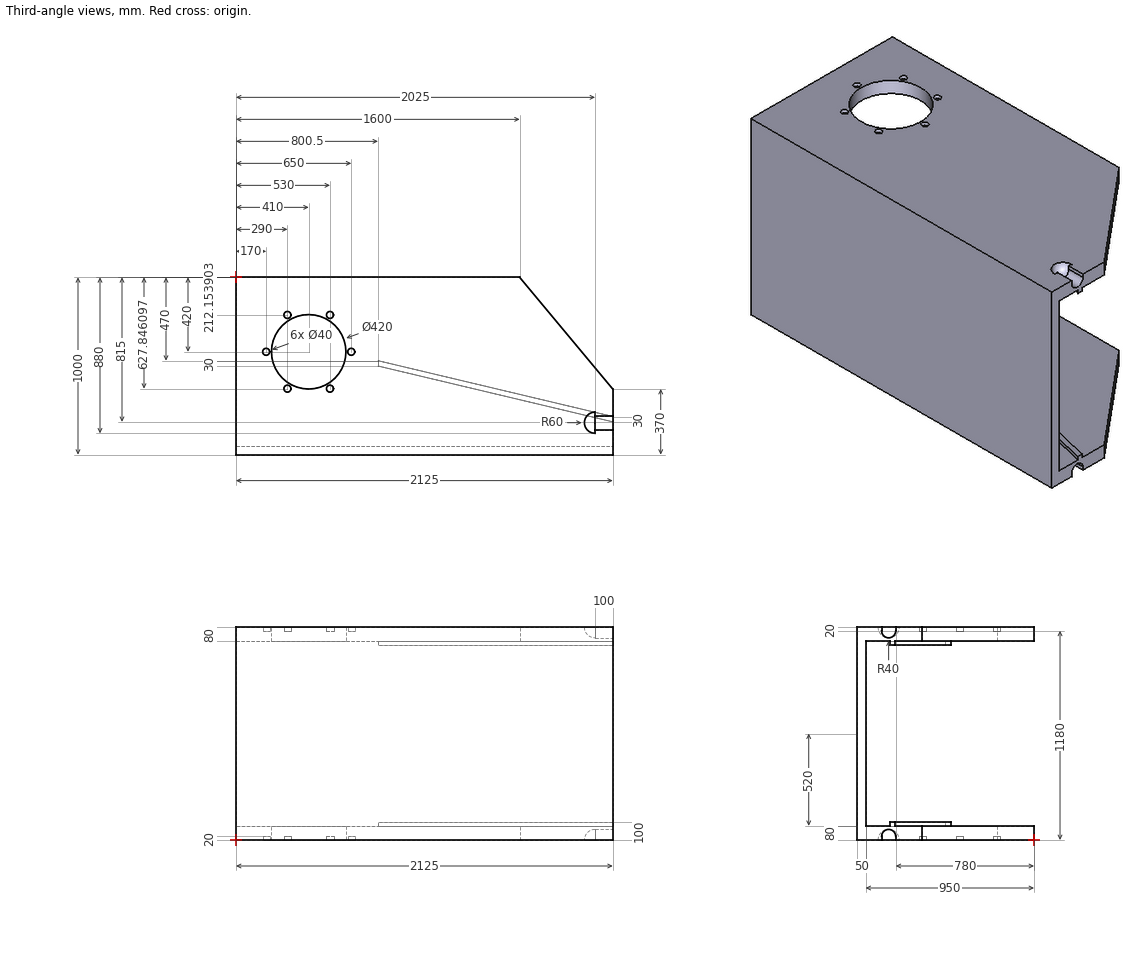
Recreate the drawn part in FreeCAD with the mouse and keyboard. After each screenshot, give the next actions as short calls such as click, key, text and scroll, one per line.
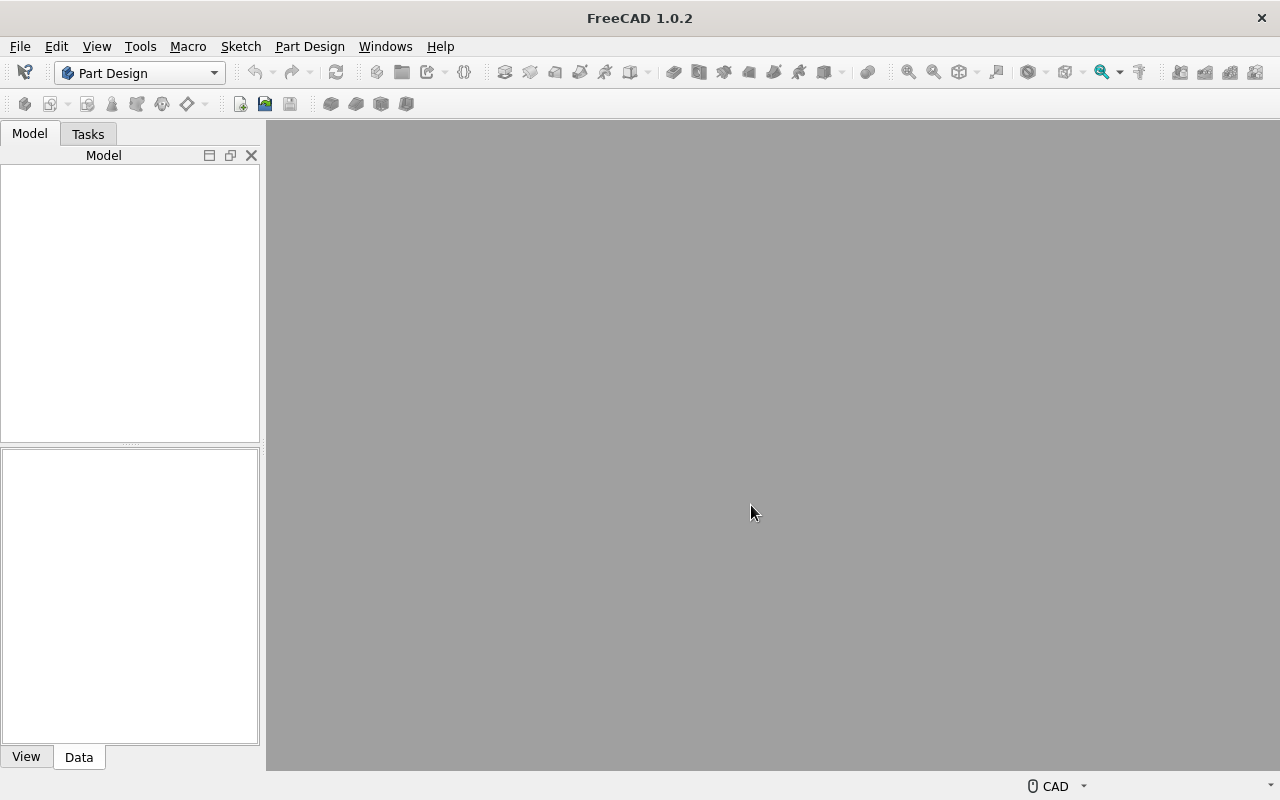
key(ctrl+n)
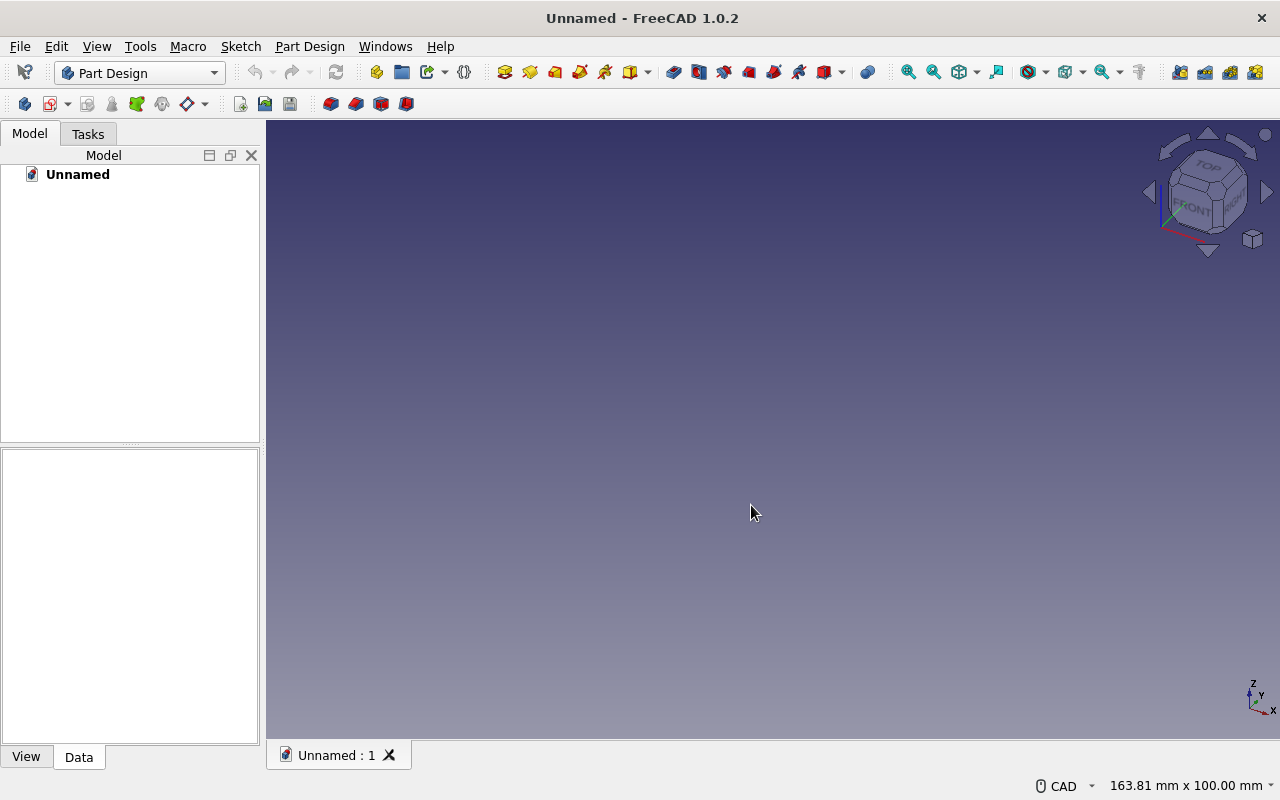
click(50, 104)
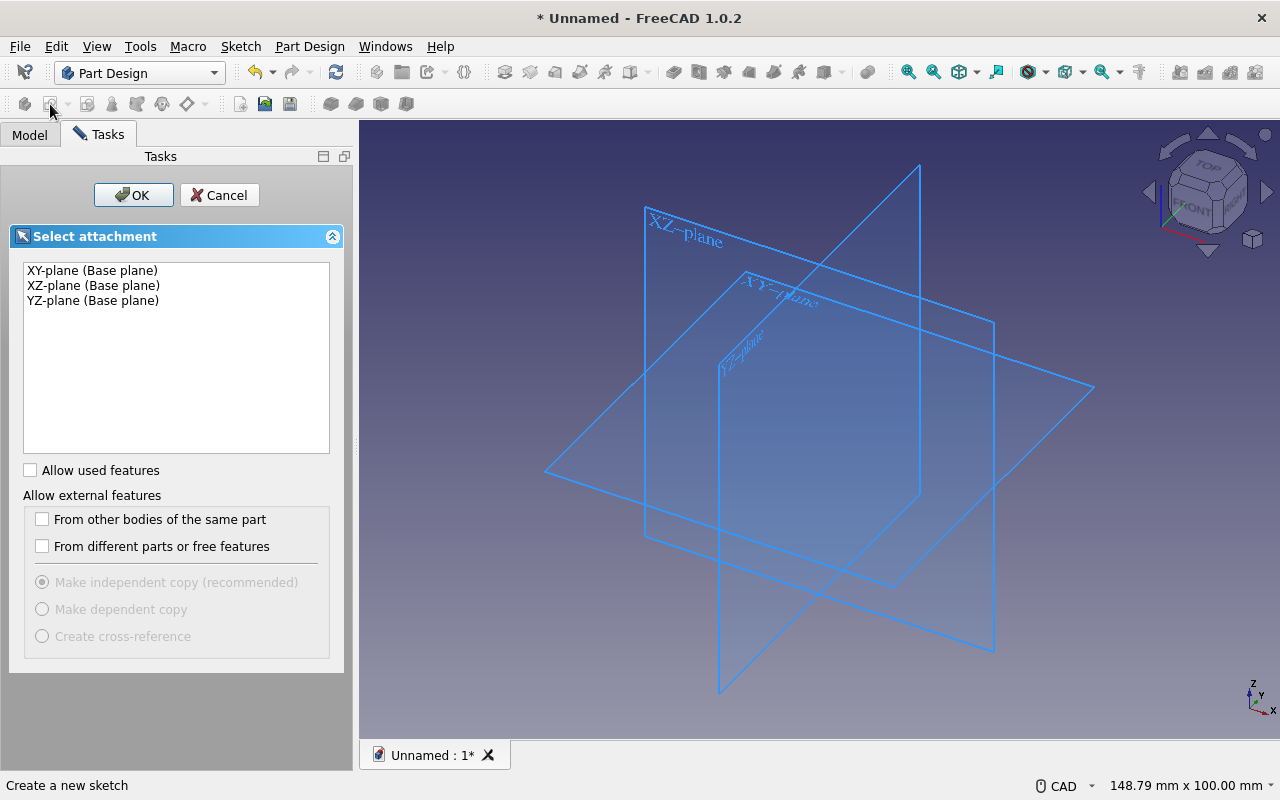
click(84, 270)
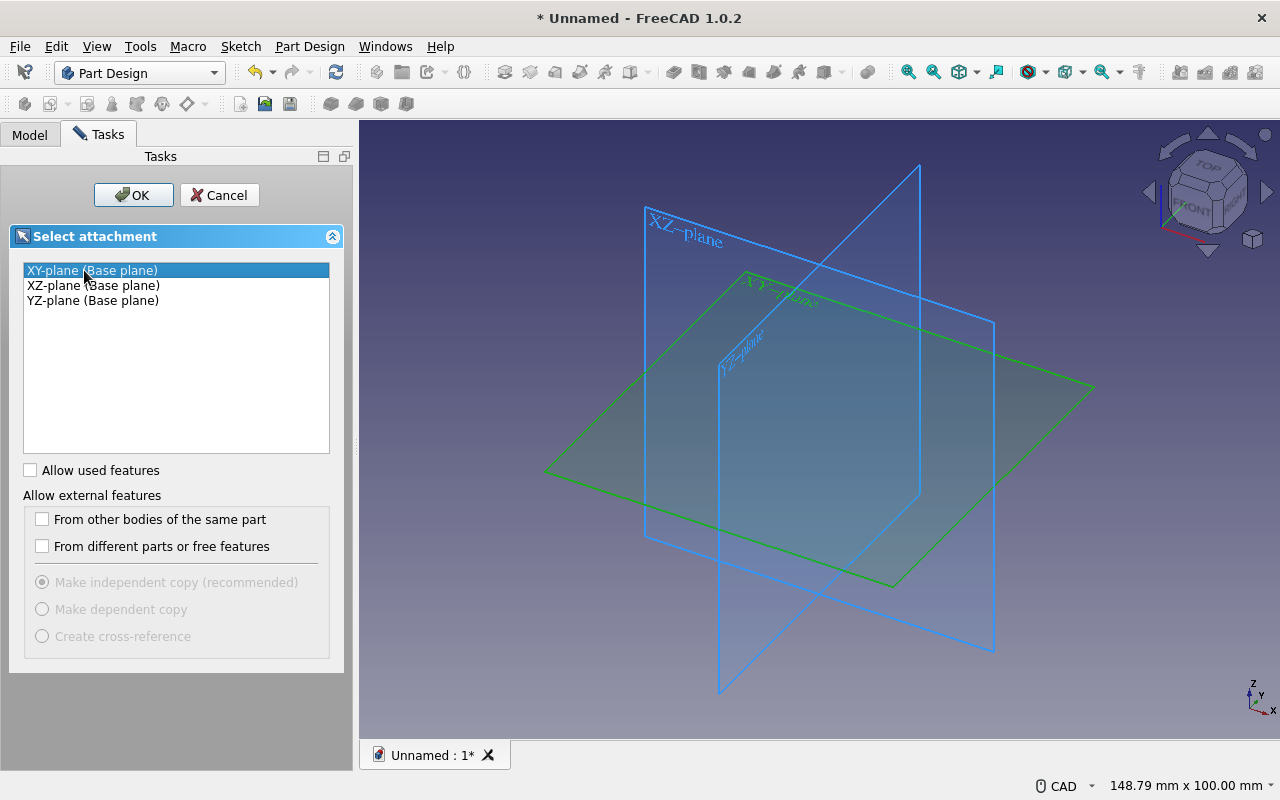
click(134, 195)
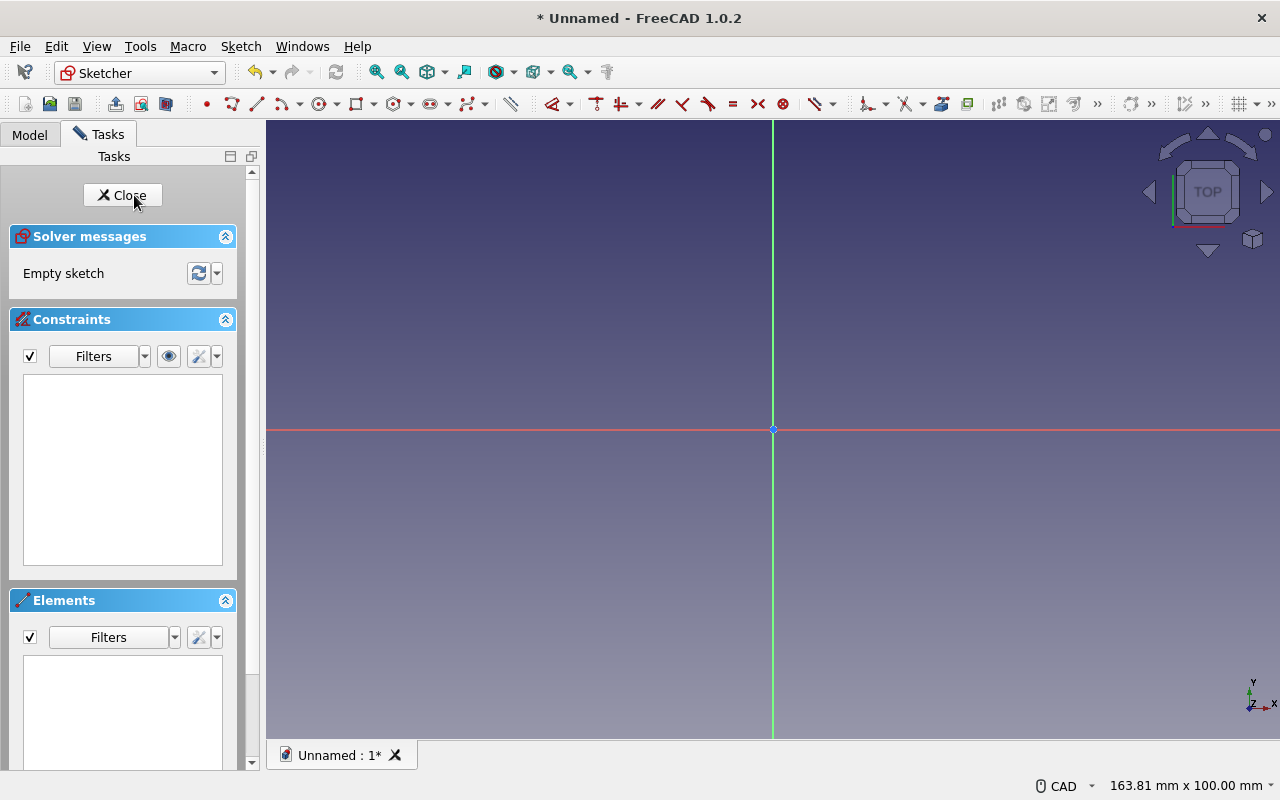
scroll(356, 267, down, 15)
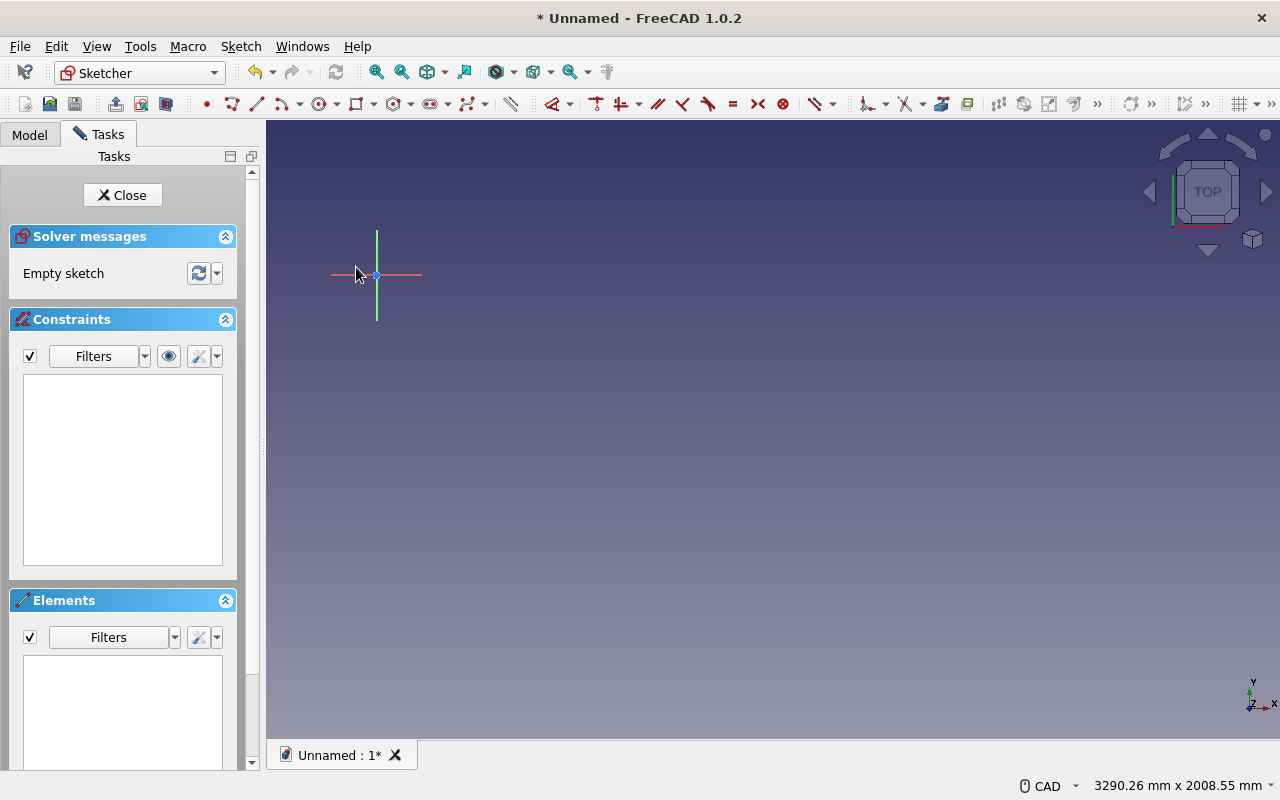
key(g)
key(m)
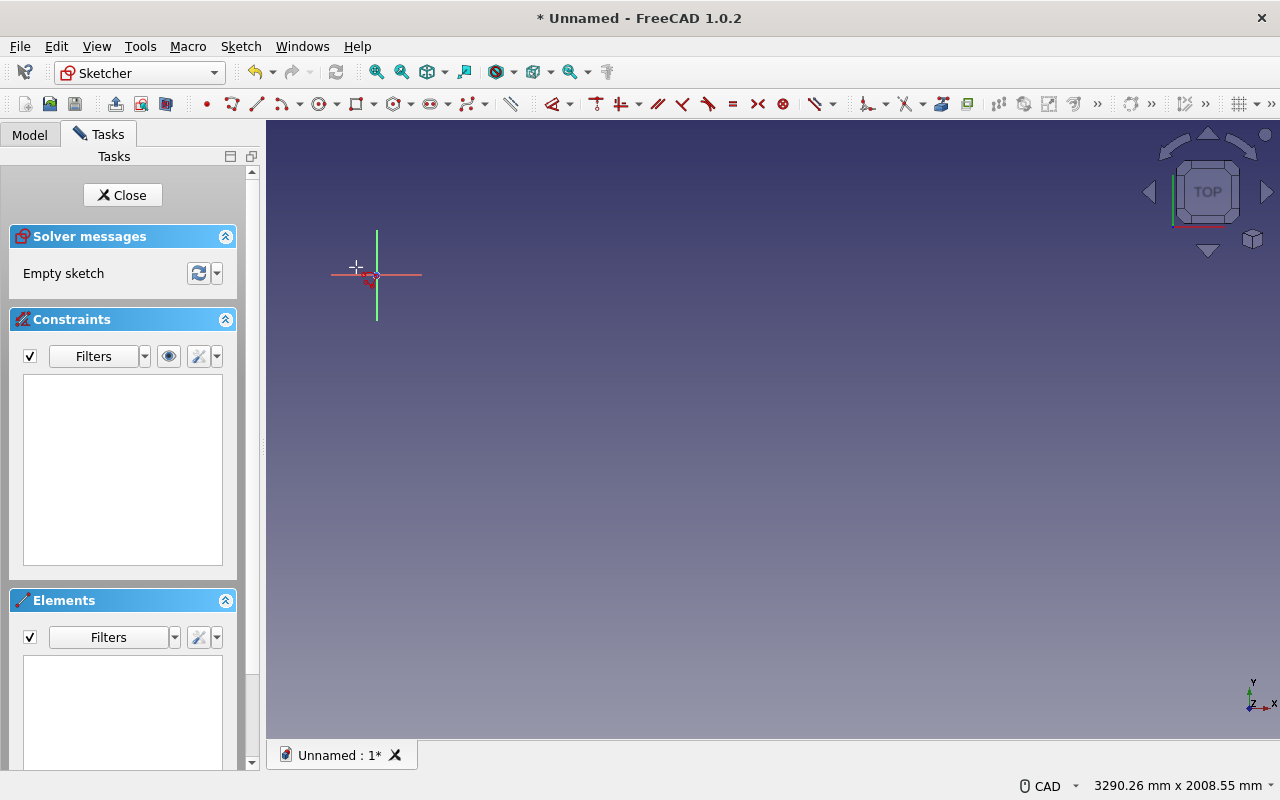
click(377, 275)
click(386, 583)
click(1032, 583)
click(1032, 469)
click(870, 284)
click(377, 275)
key(Escape)
key(Escape)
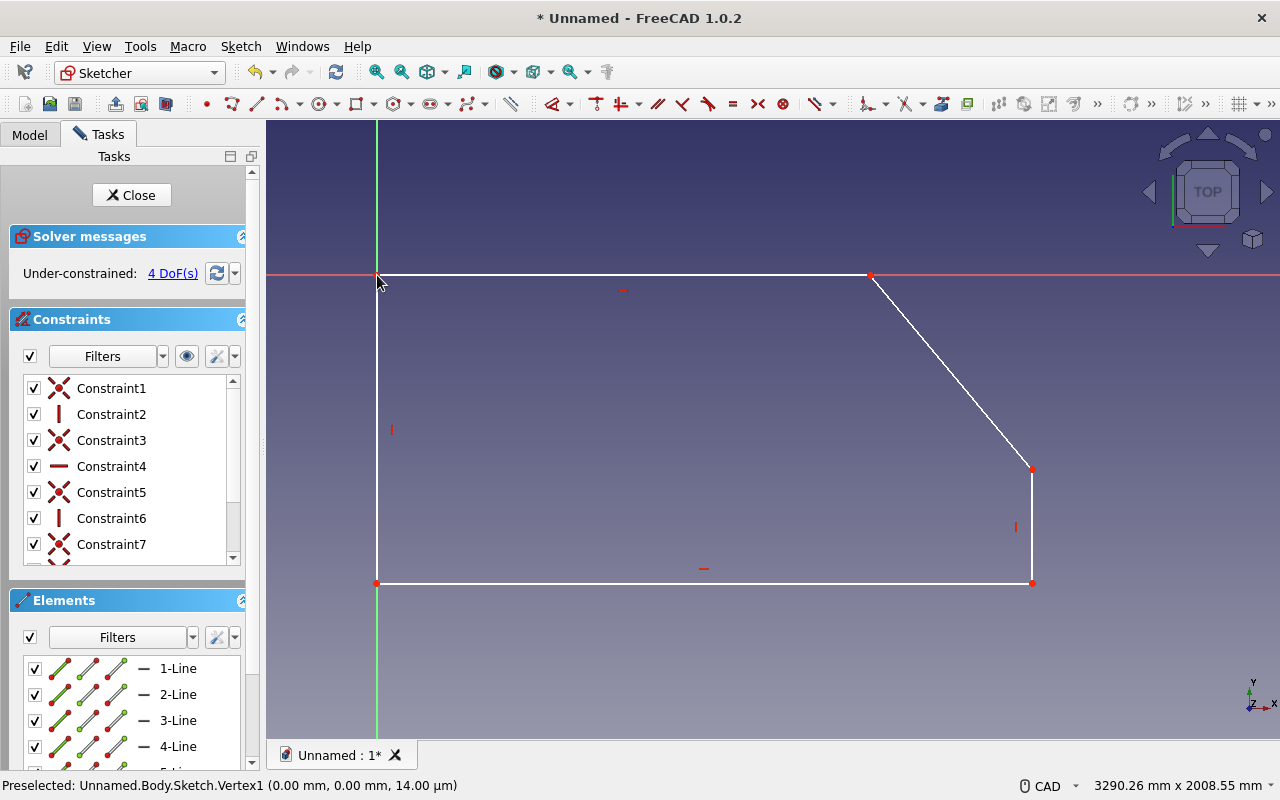
key(d)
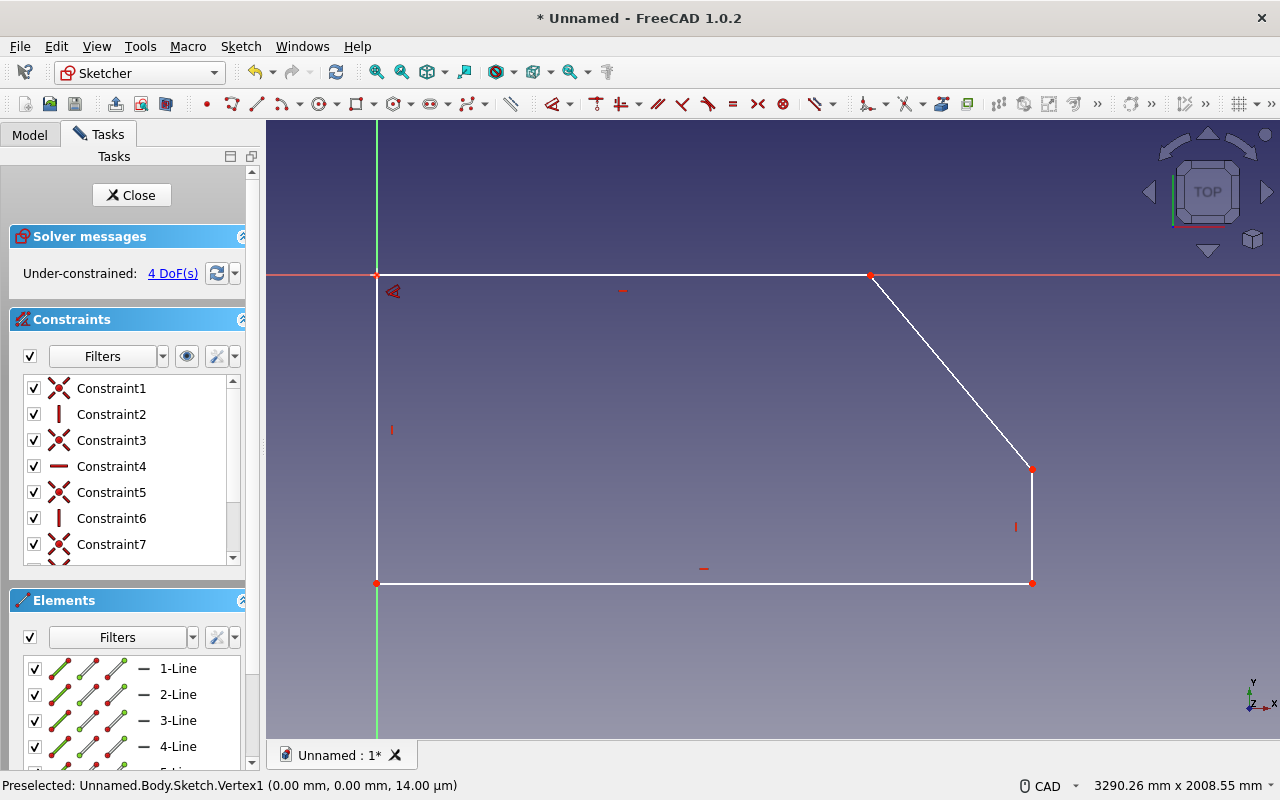
click(1032, 550)
click(1066, 527)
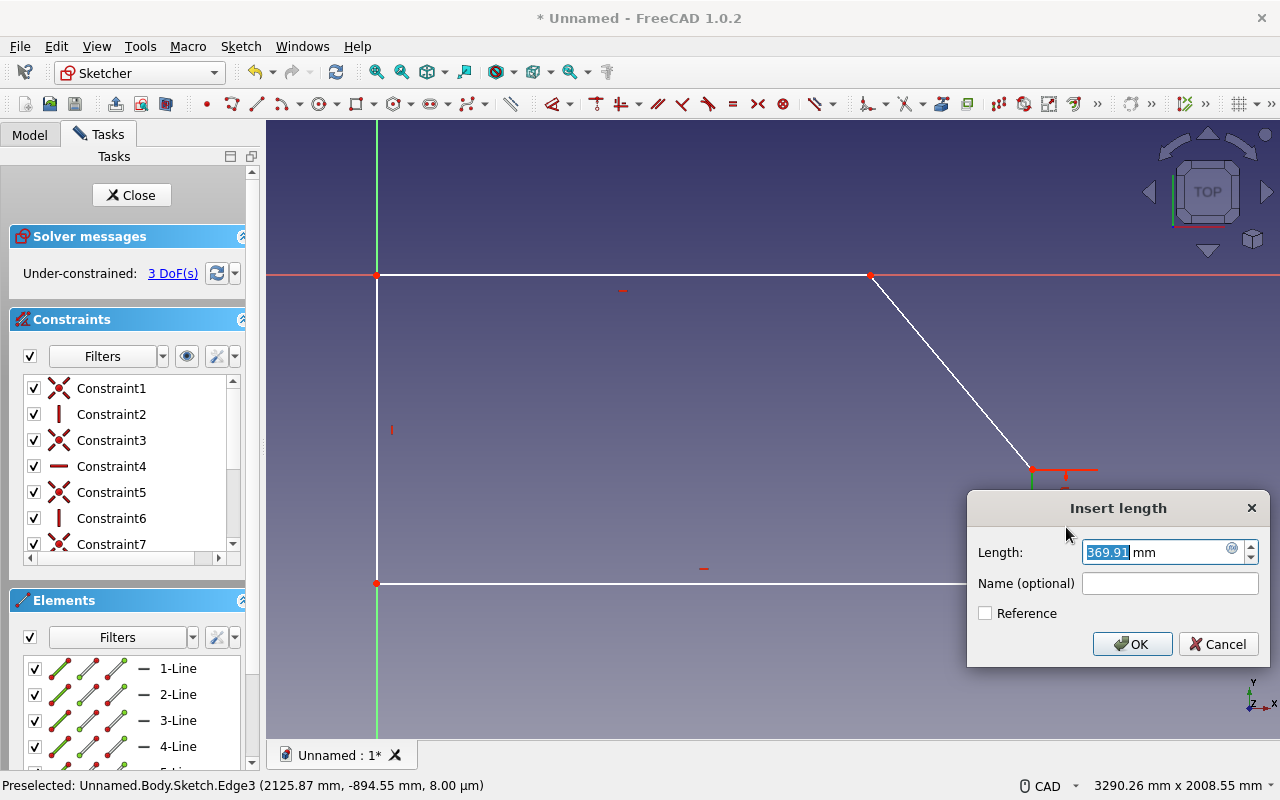
text(370)
key(Return)